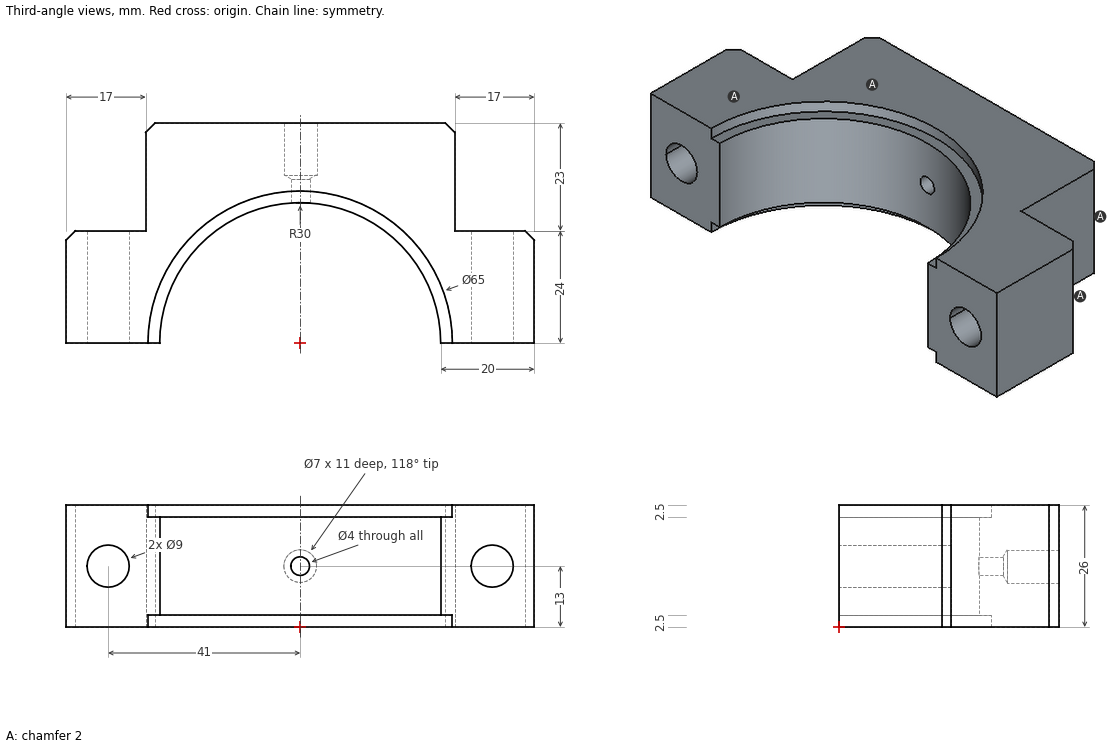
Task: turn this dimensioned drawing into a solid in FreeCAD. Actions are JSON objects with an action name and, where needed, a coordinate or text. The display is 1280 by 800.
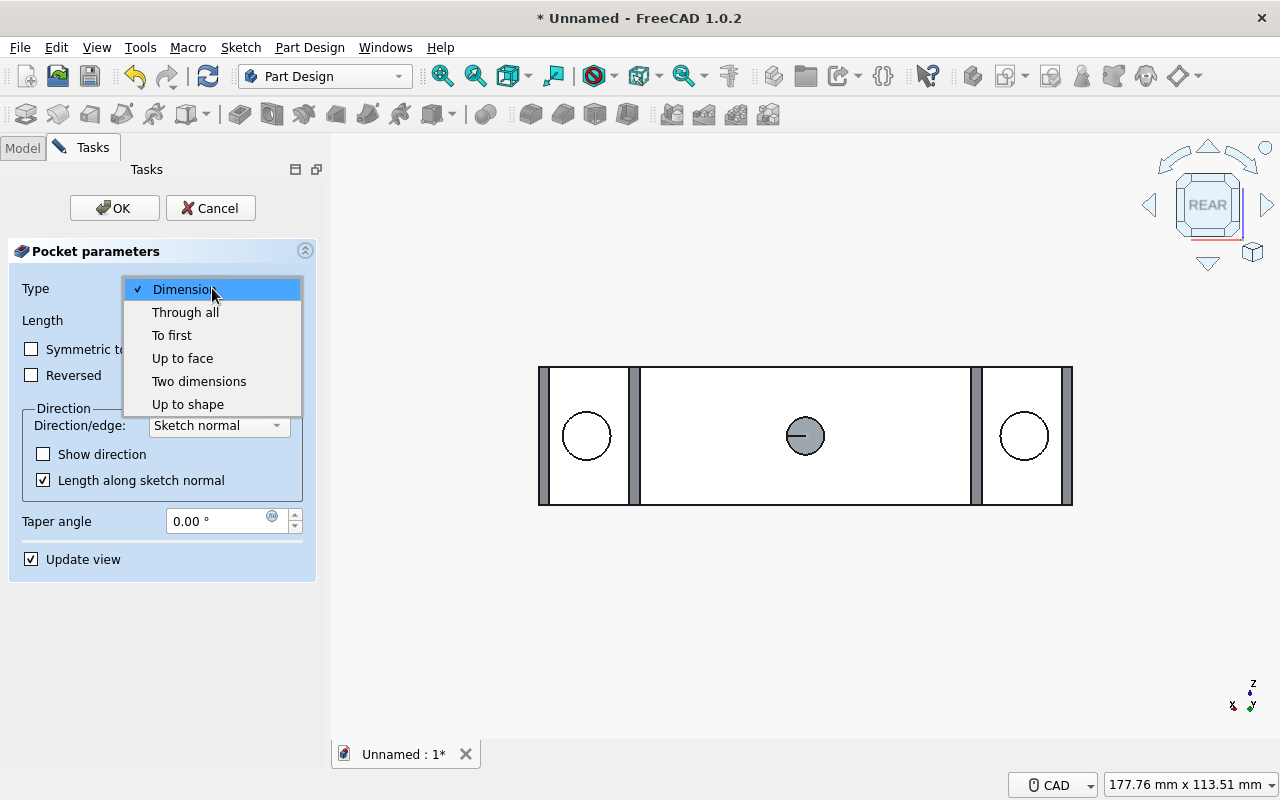
{"action": "left_click", "coordinate": [212, 312]}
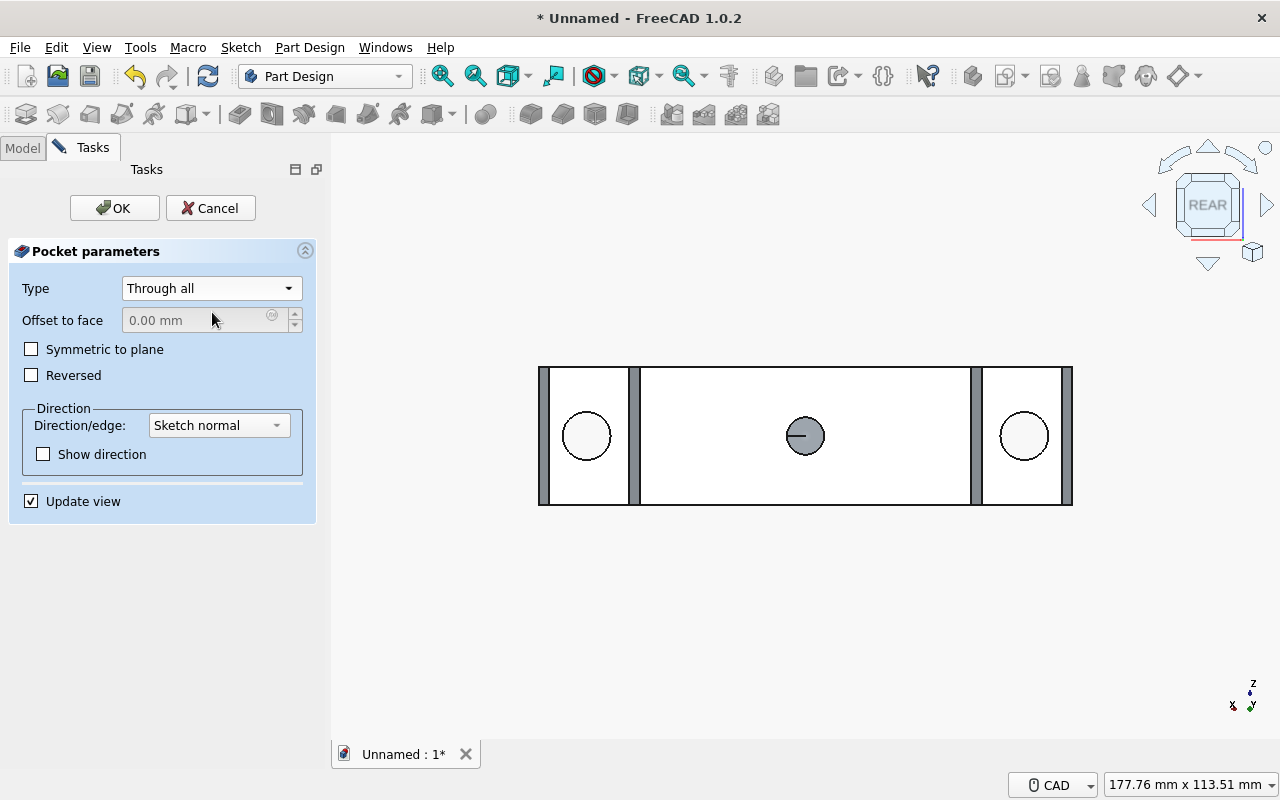
{"action": "left_click", "coordinate": [115, 208]}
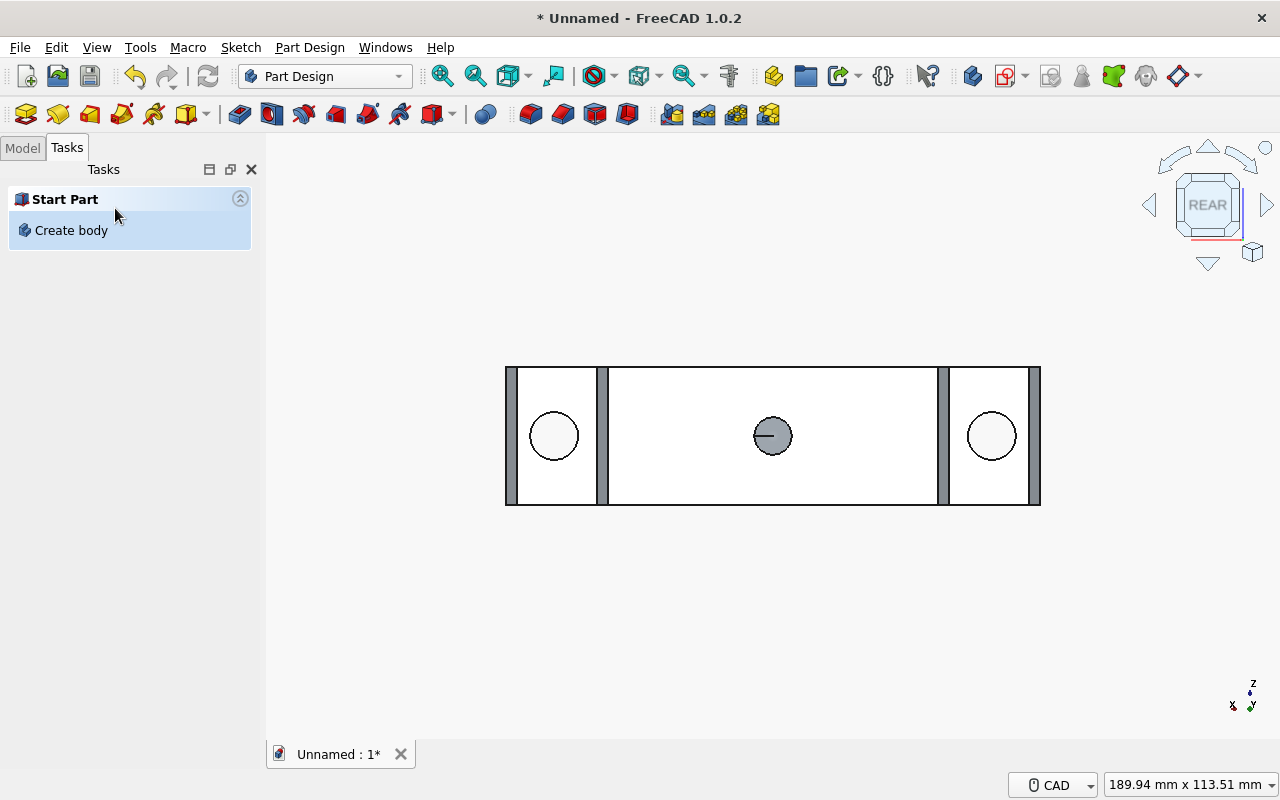
{"action": "key", "text": "0"}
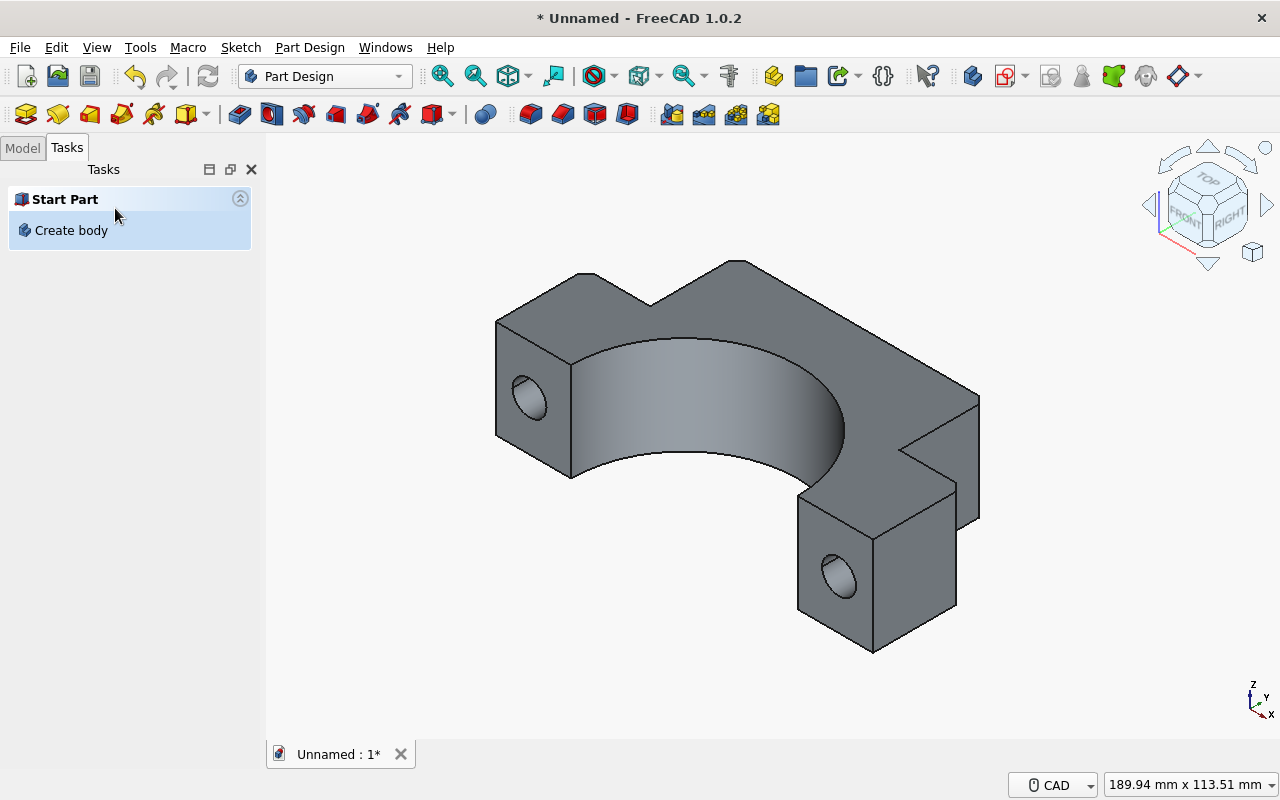
{"action": "left_click", "coordinate": [878, 380]}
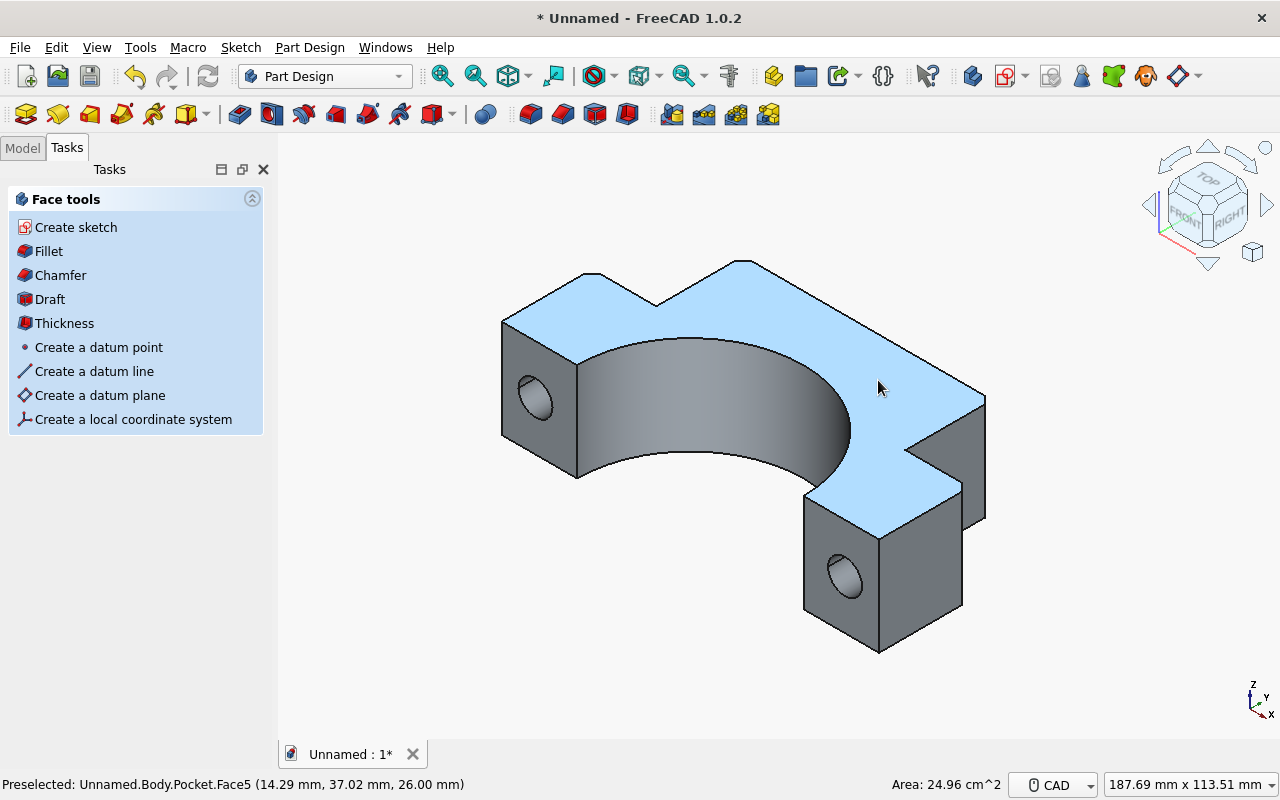
{"action": "left_click", "coordinate": [1006, 76]}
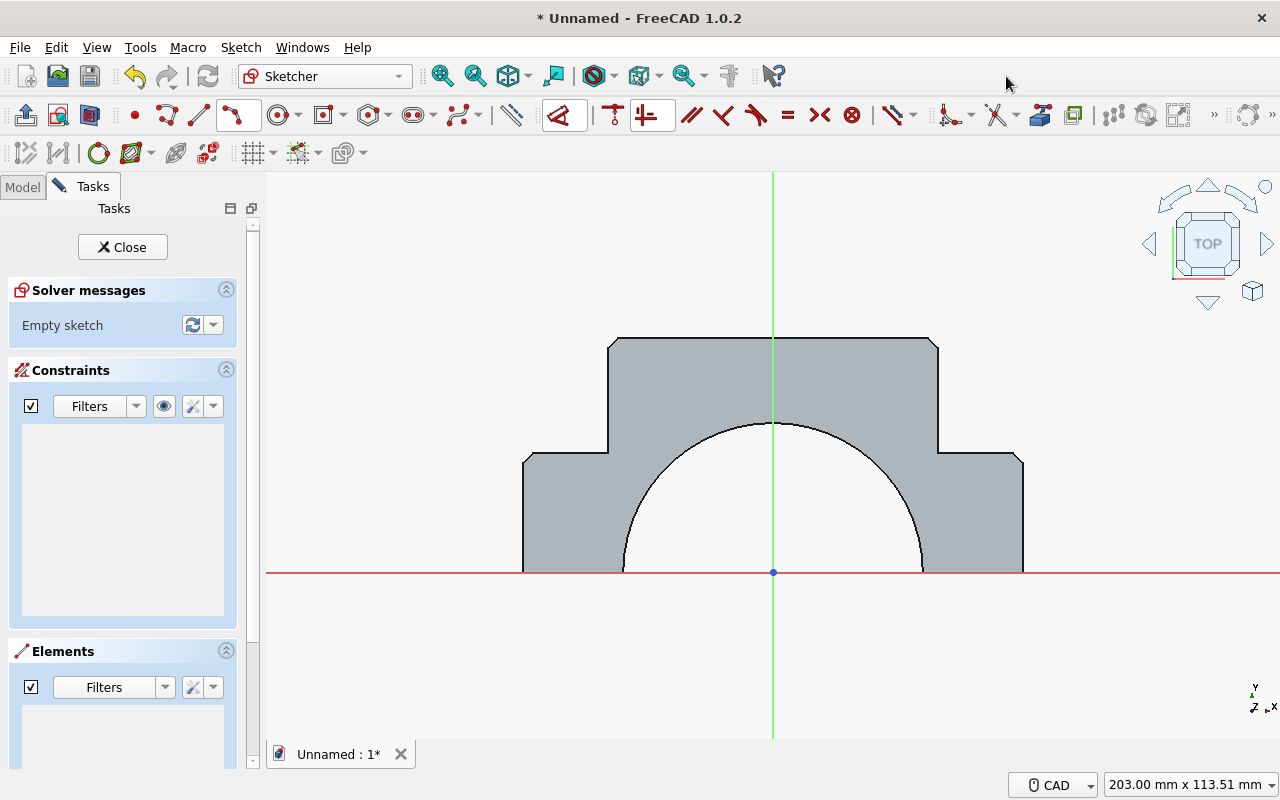
{"action": "scroll", "coordinate": [395, 200], "scroll_direction": "down", "scroll_amount": 1}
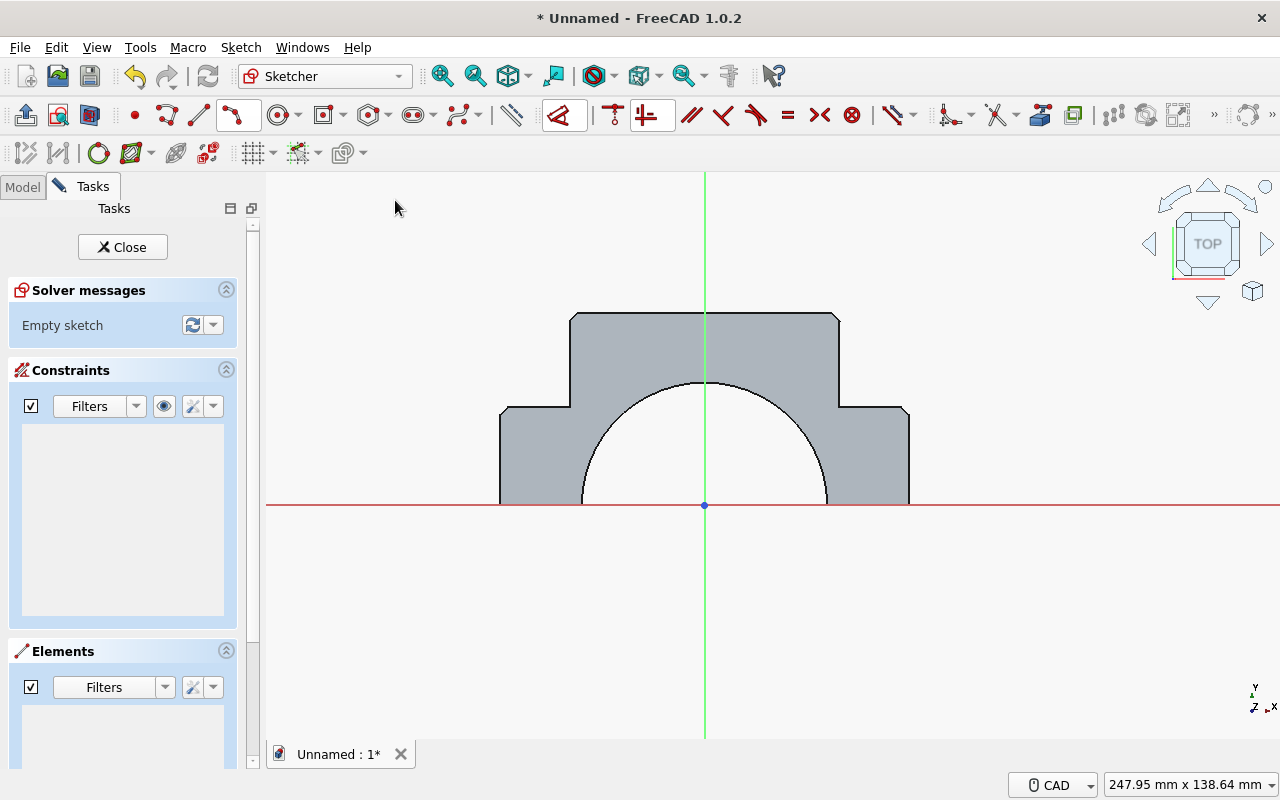
{"action": "scroll", "coordinate": [705, 607], "scroll_direction": "up", "scroll_amount": 2}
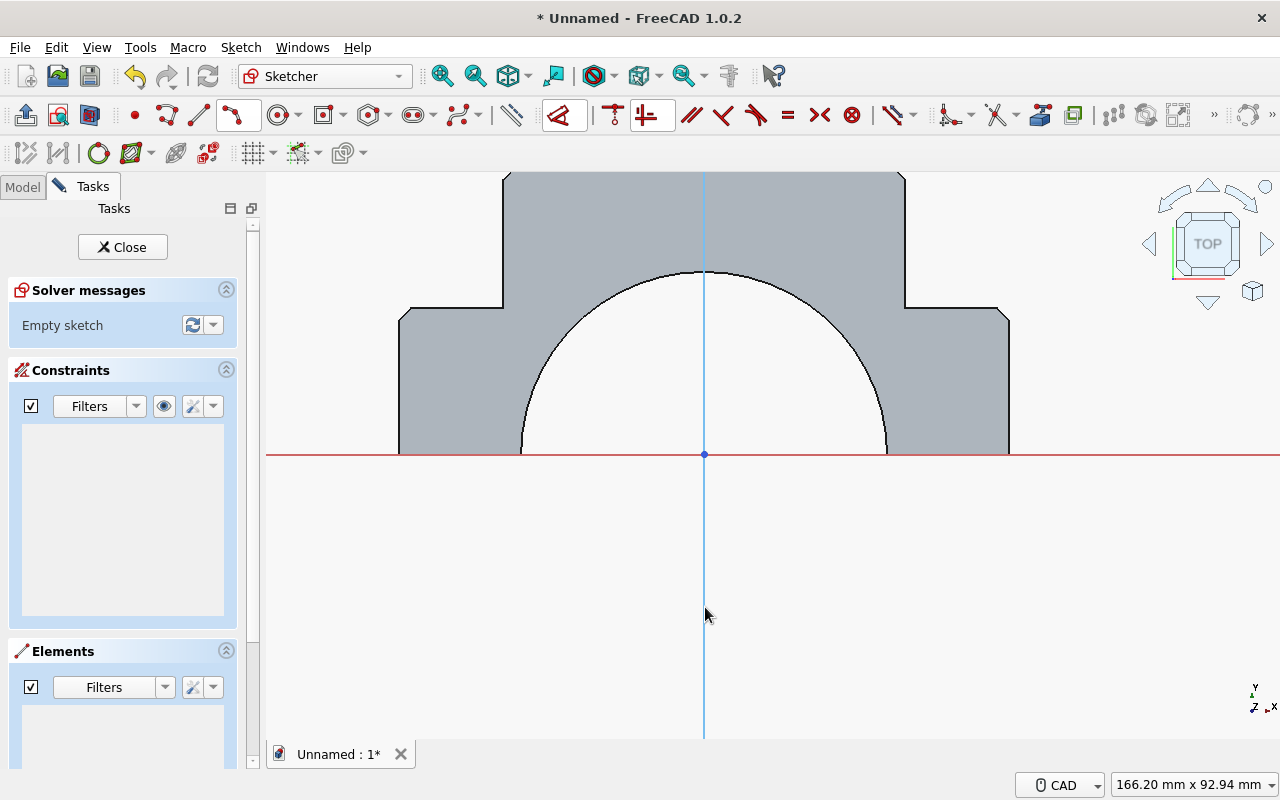
{"action": "left_click", "coordinate": [278, 116]}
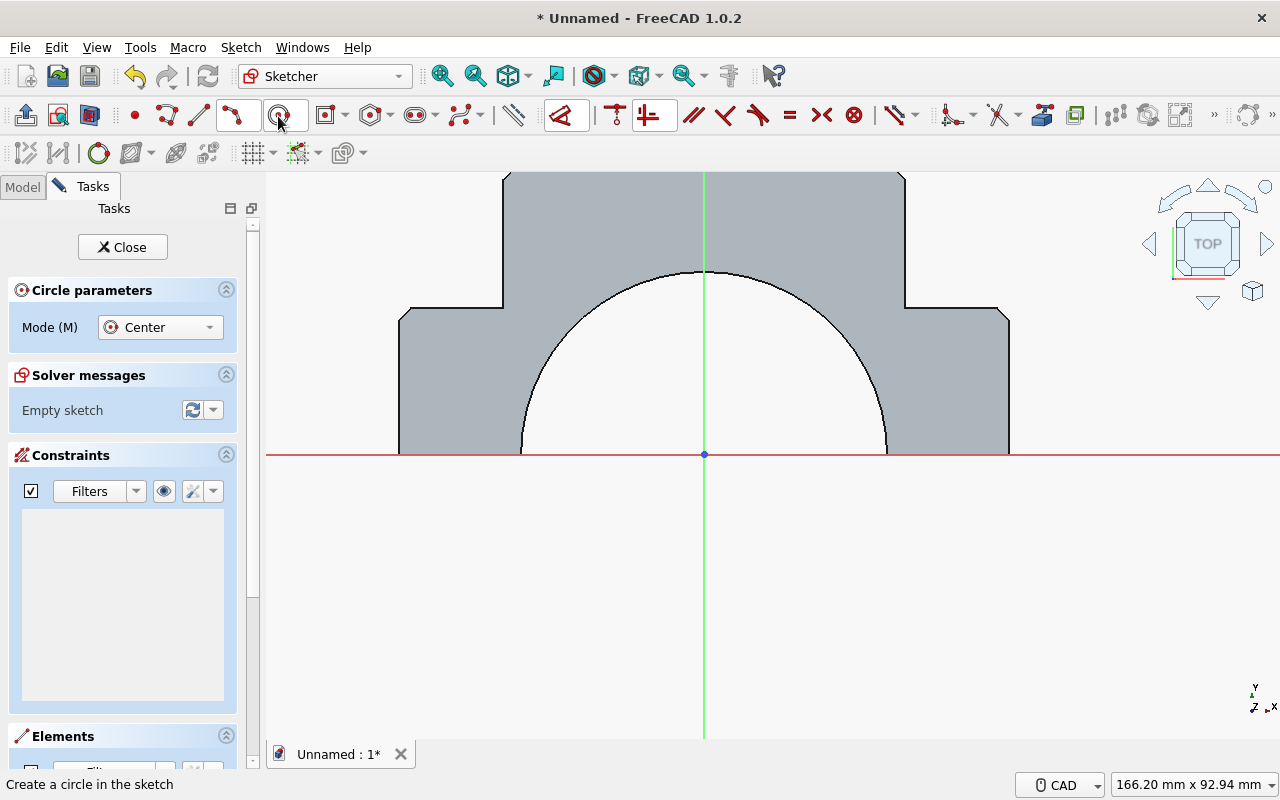
{"action": "left_click", "coordinate": [704, 455]}
{"action": "left_click", "coordinate": [844, 315]}
{"action": "key", "text": "Escape"}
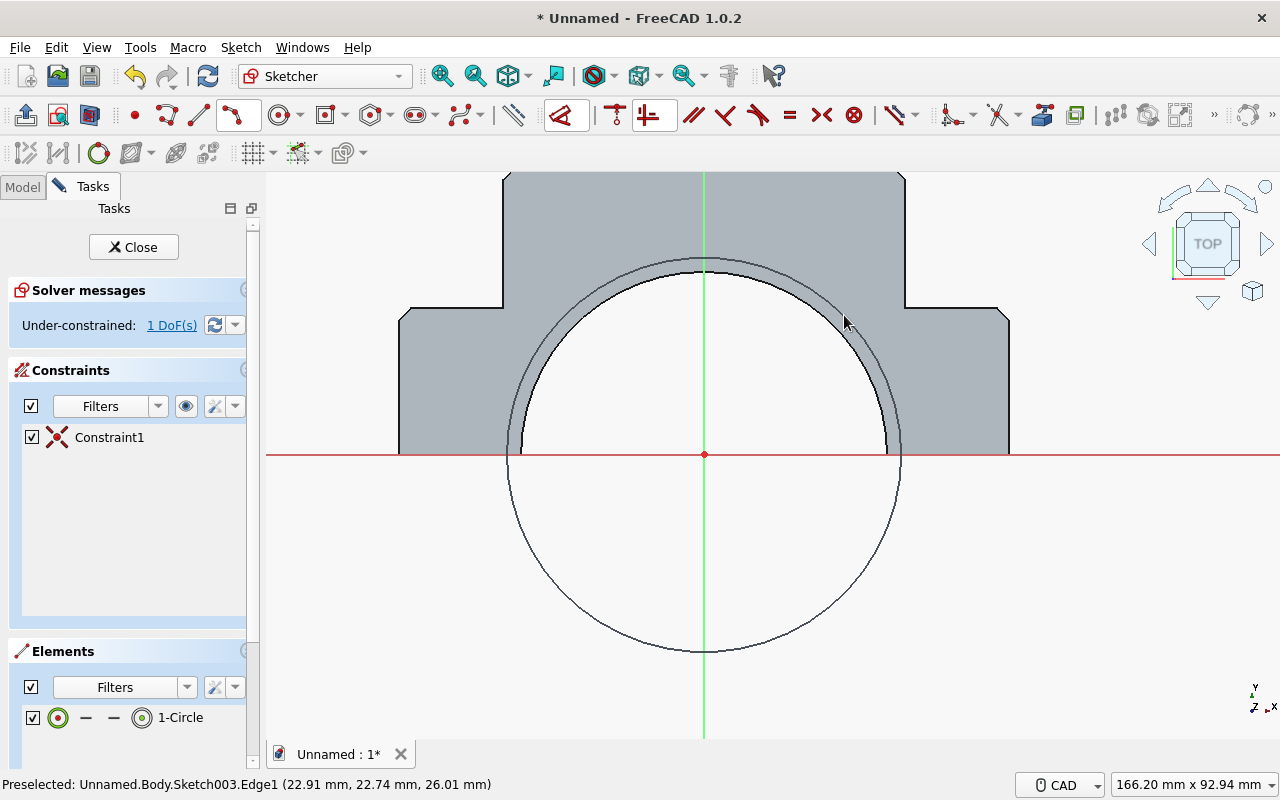
{"action": "left_click", "coordinate": [843, 315]}